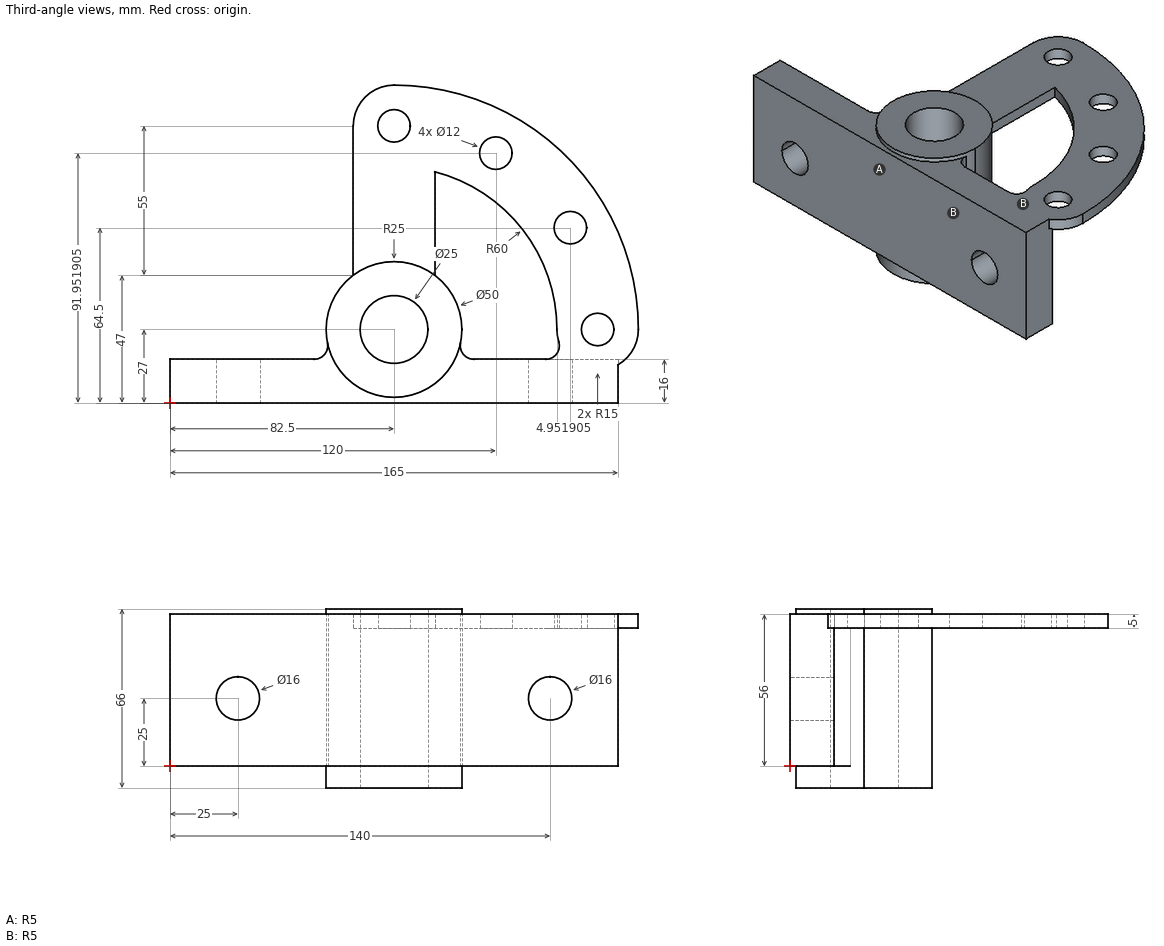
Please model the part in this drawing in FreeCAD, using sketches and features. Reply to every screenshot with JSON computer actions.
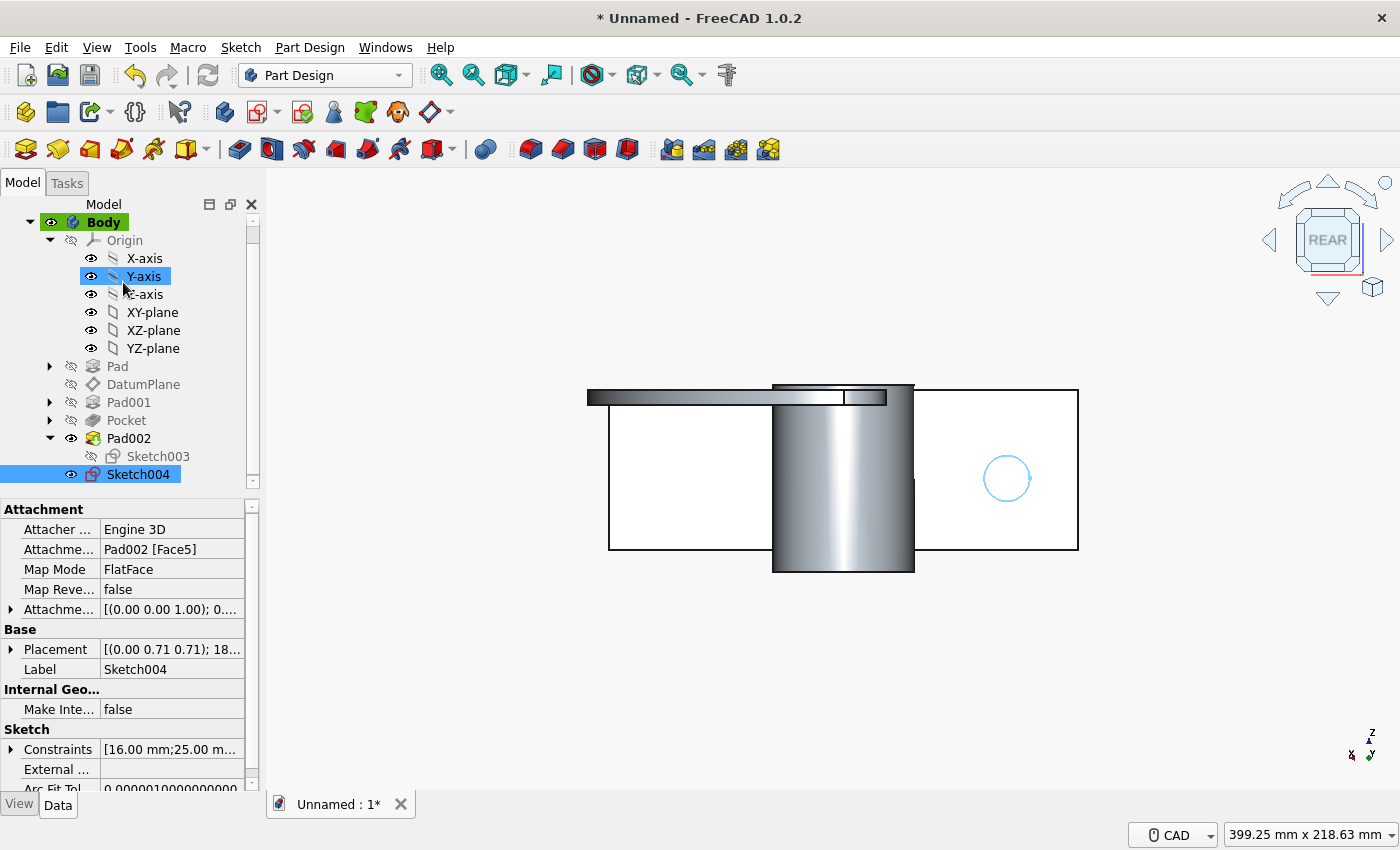
{"action": "left_click", "coordinate": [240, 150]}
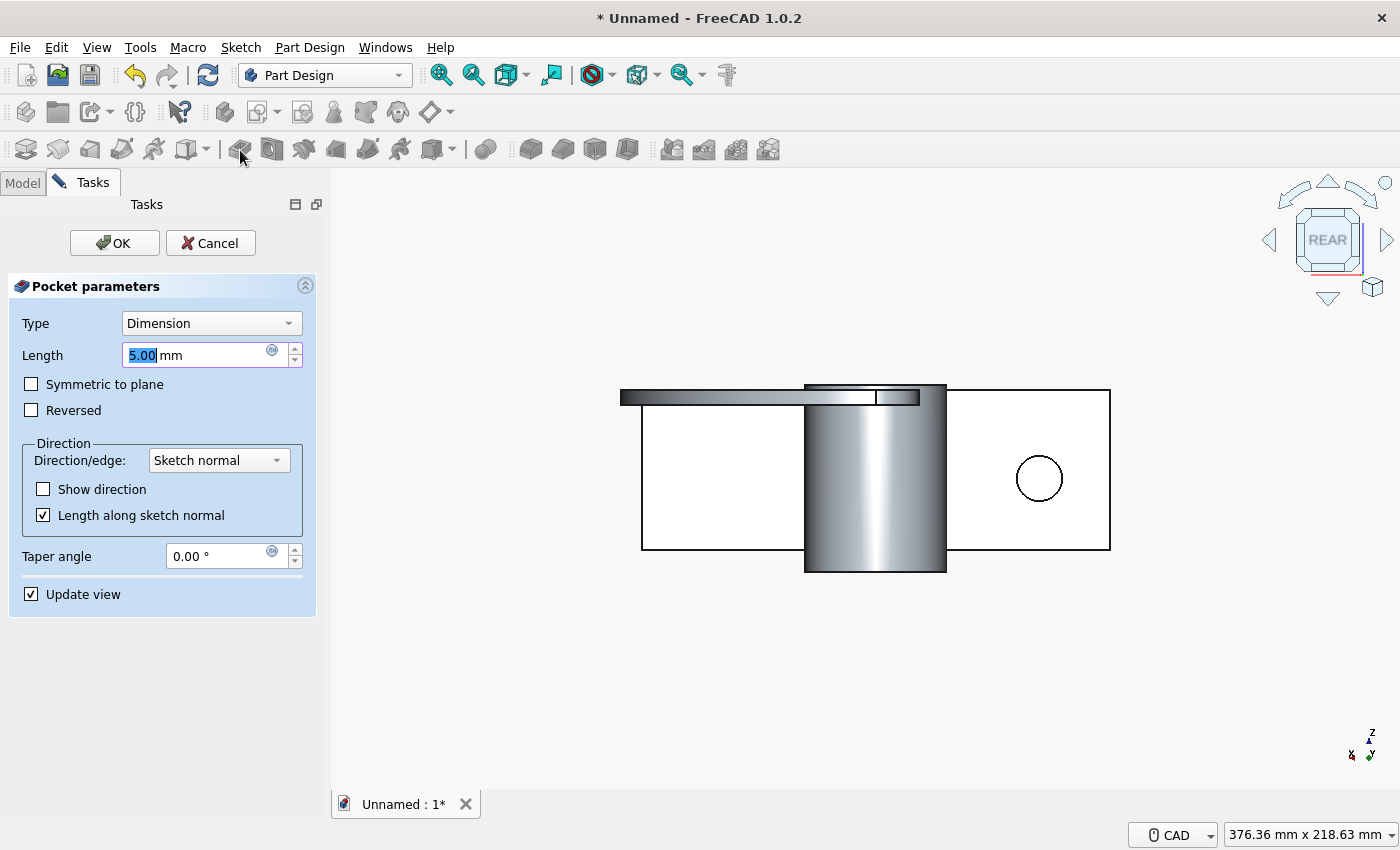
{"action": "left_click", "coordinate": [212, 324]}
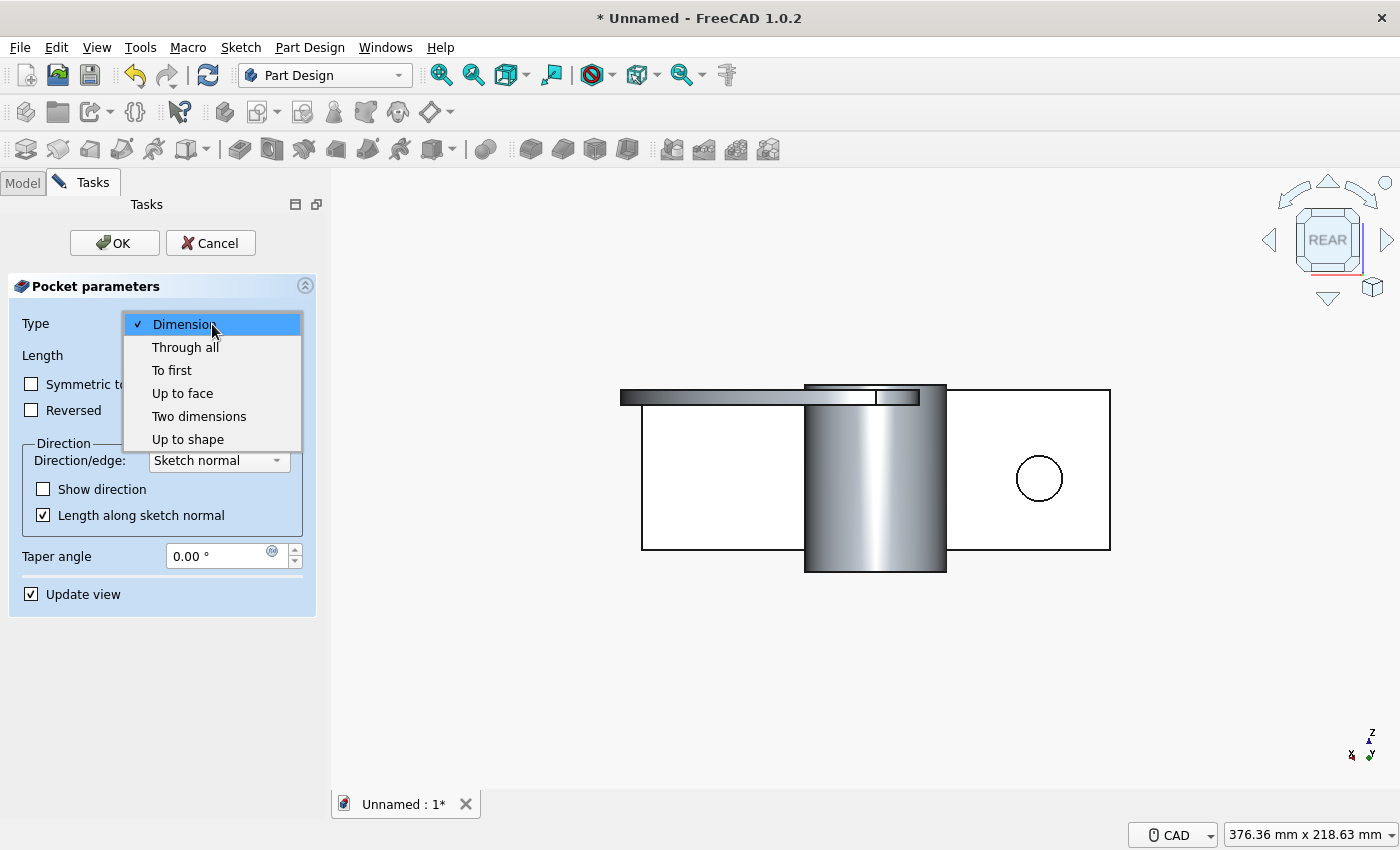
{"action": "left_click", "coordinate": [212, 348]}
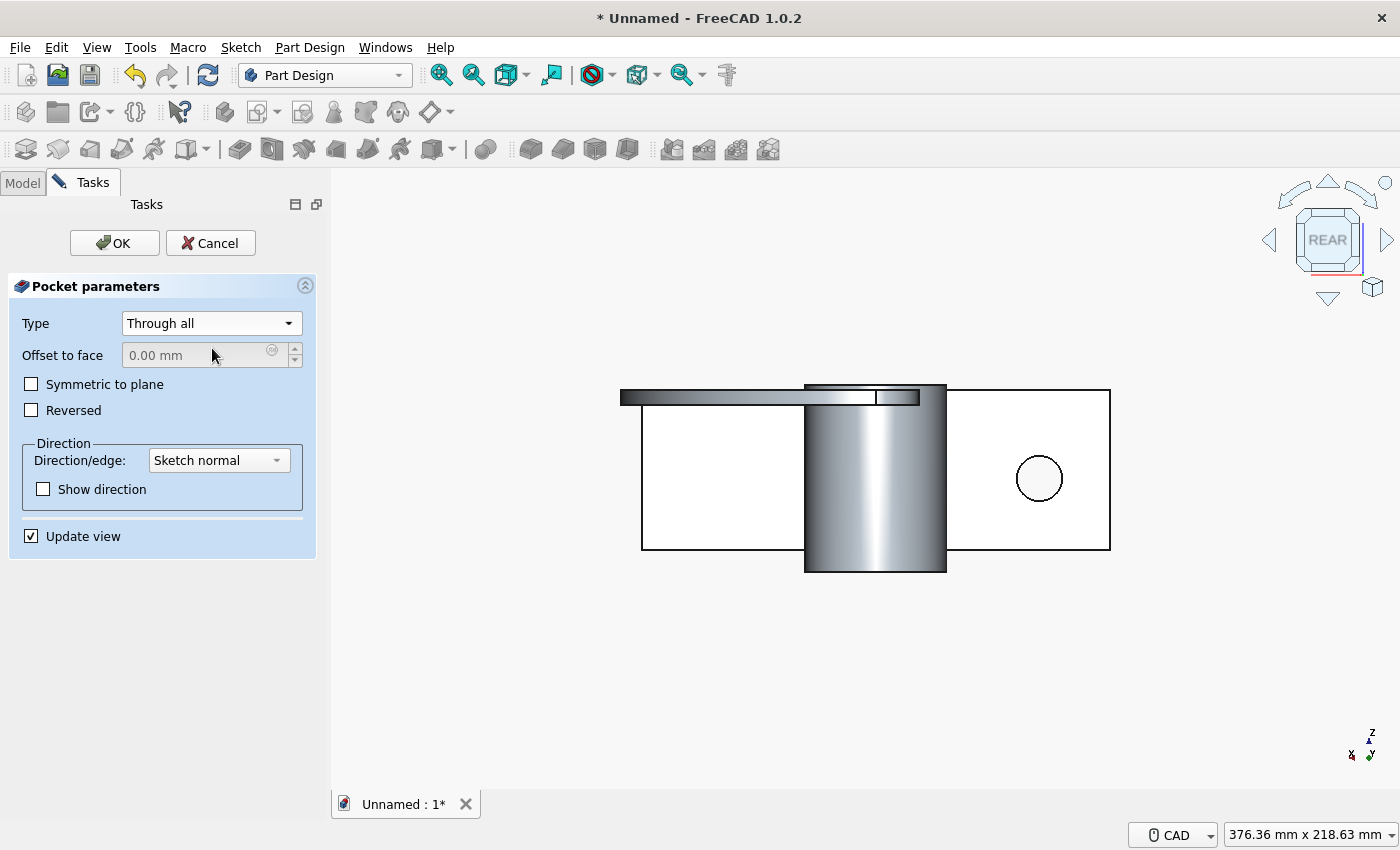
{"action": "left_click", "coordinate": [115, 243]}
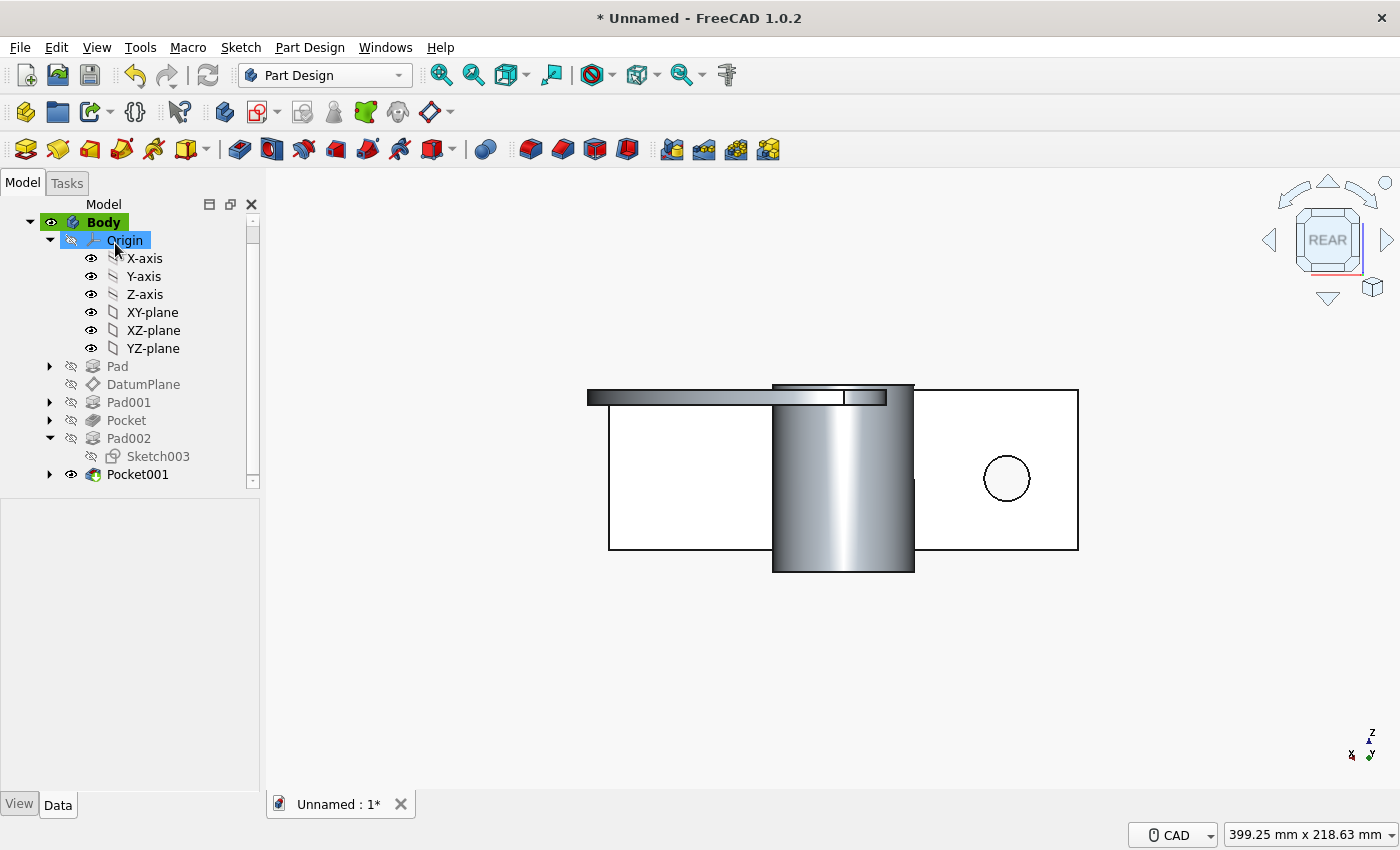
{"action": "left_click", "coordinate": [442, 76]}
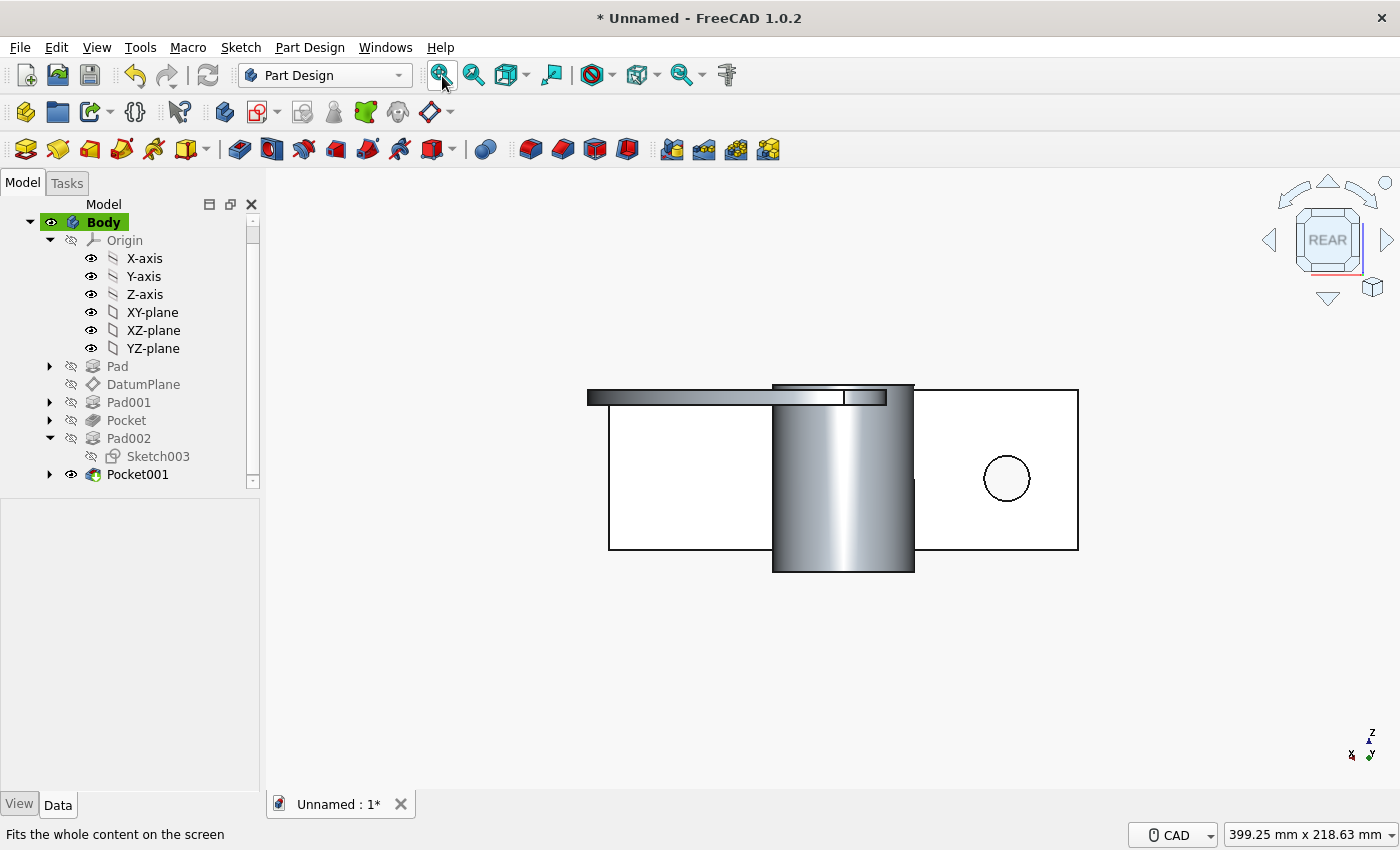
{"action": "left_click", "coordinate": [695, 469]}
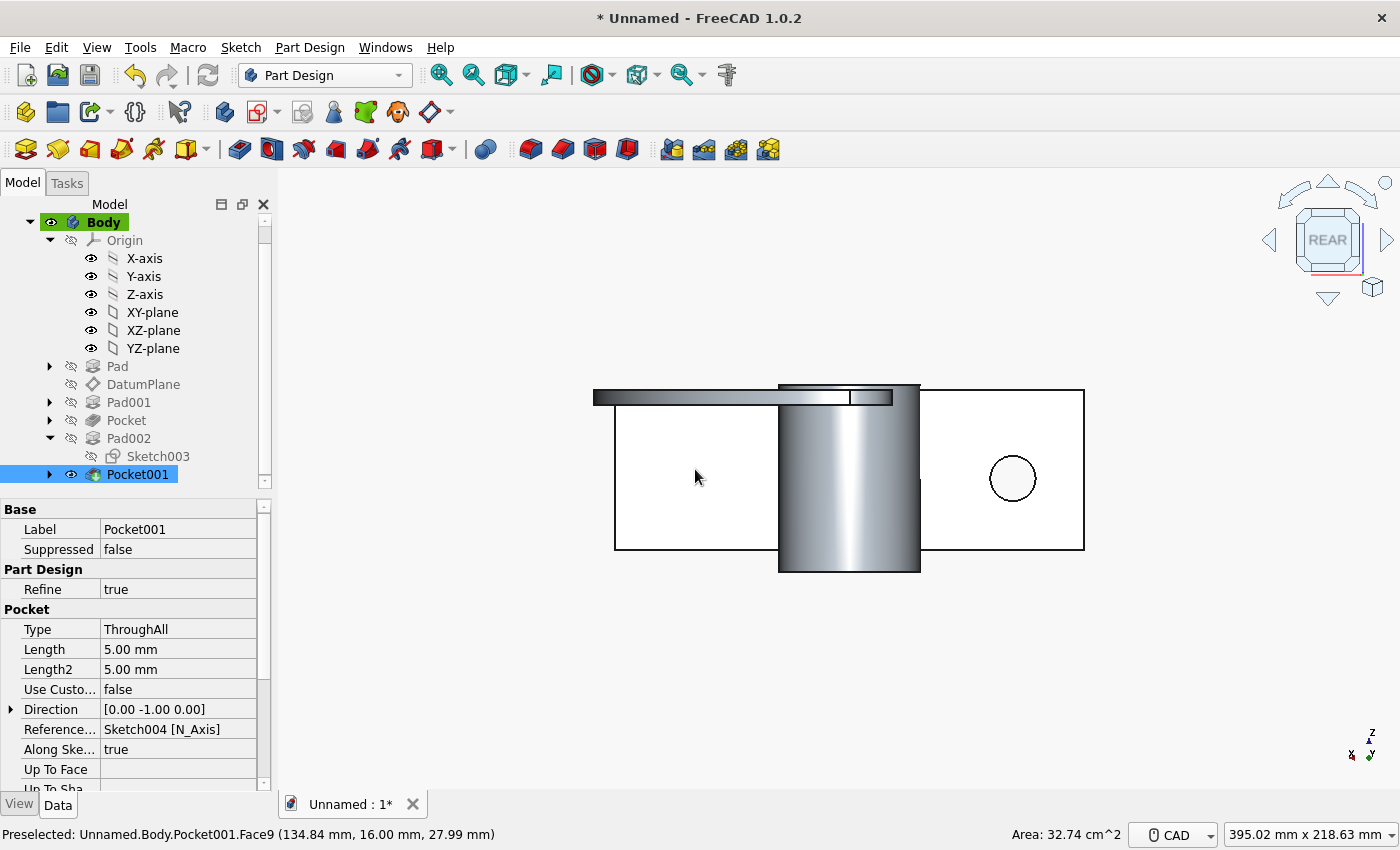
{"action": "left_click", "coordinate": [258, 112]}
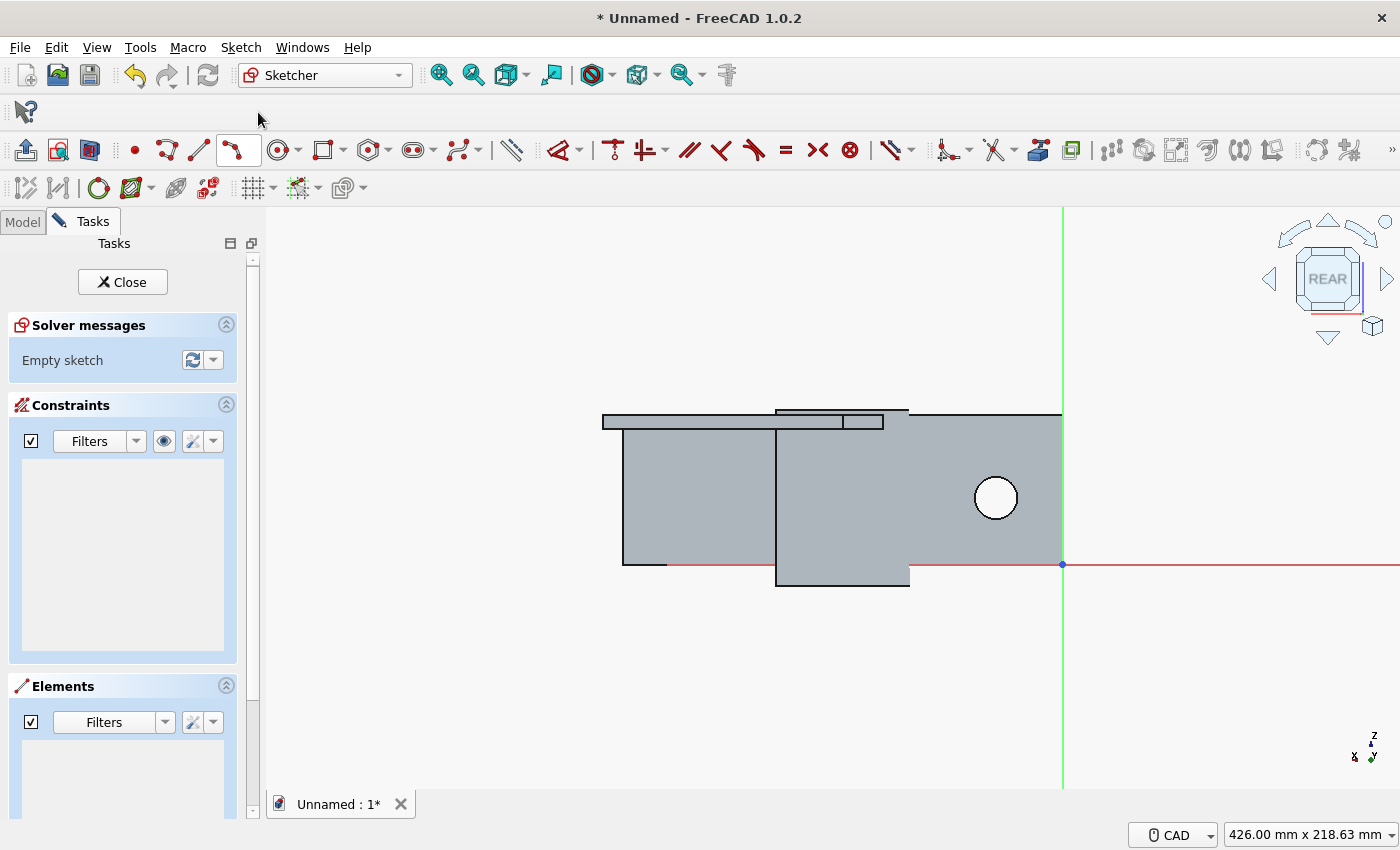
{"action": "left_click", "coordinate": [90, 150]}